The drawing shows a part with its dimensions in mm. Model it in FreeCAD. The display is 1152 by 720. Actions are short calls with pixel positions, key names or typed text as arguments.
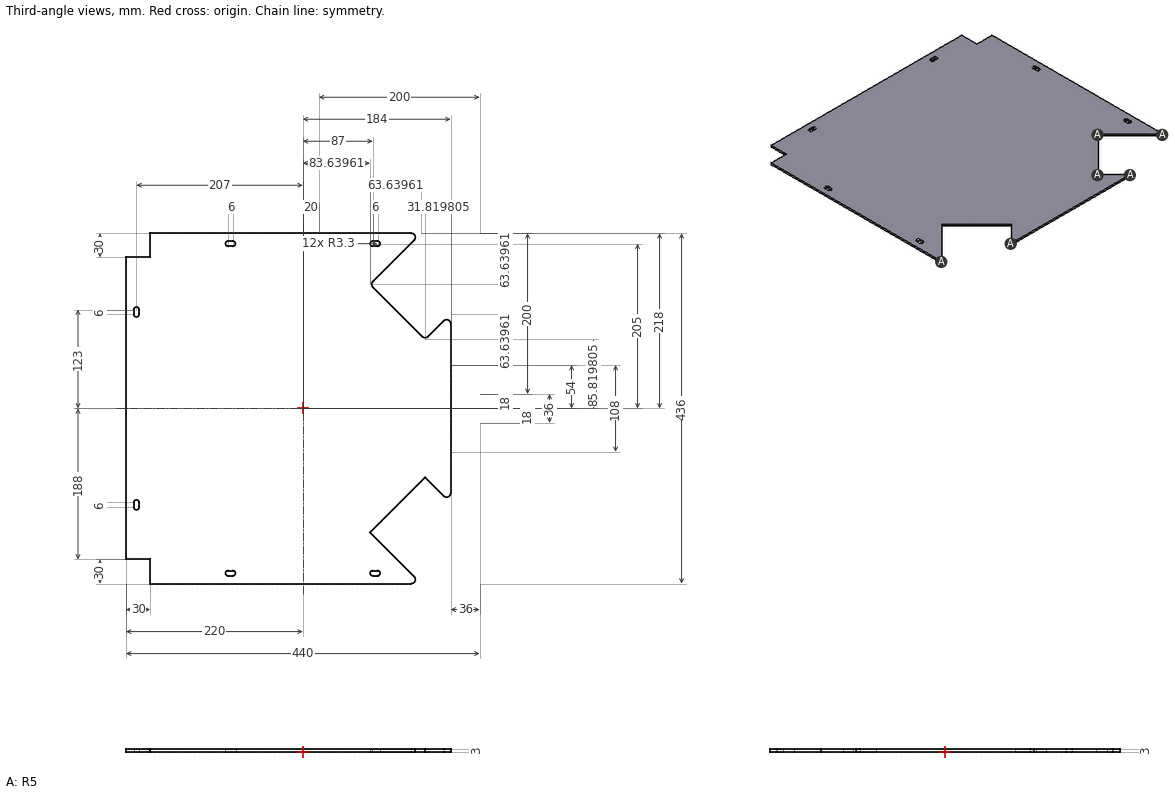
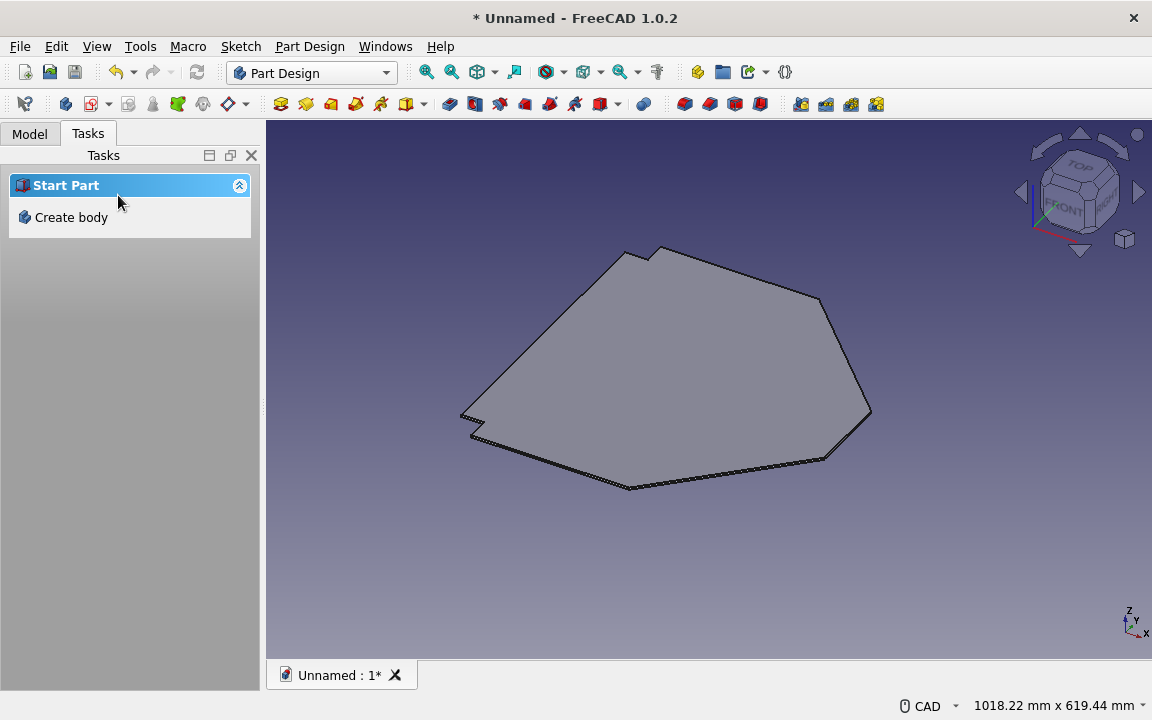
click(695, 383)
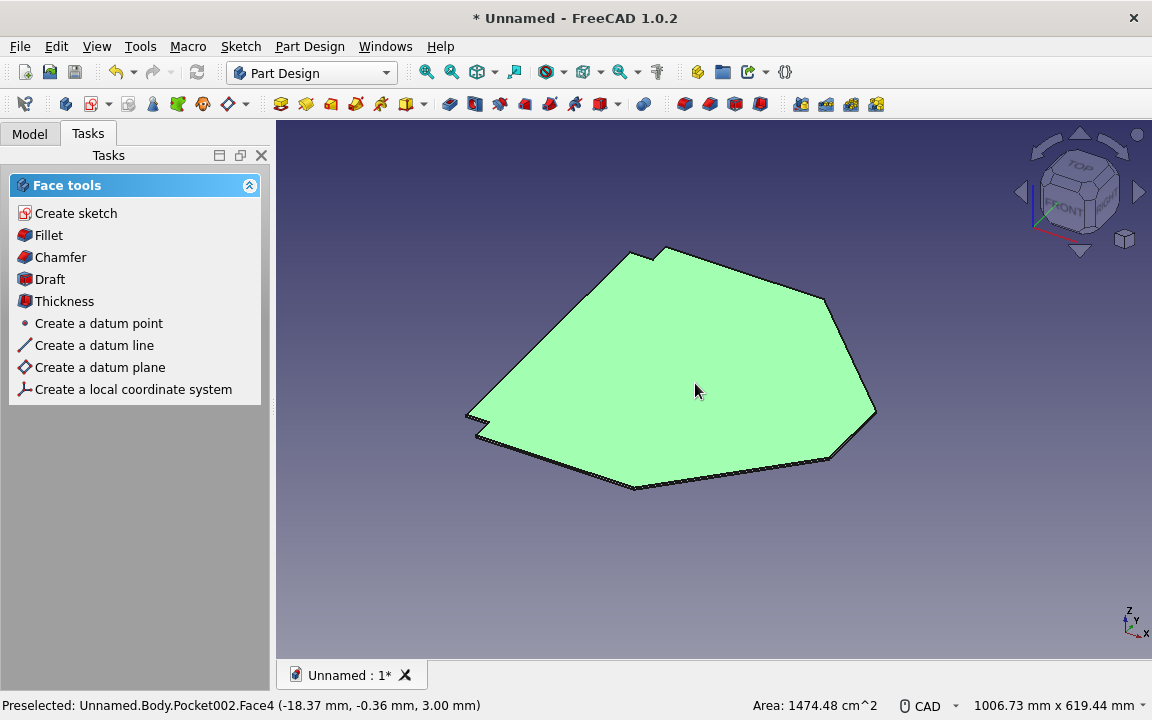
click(90, 104)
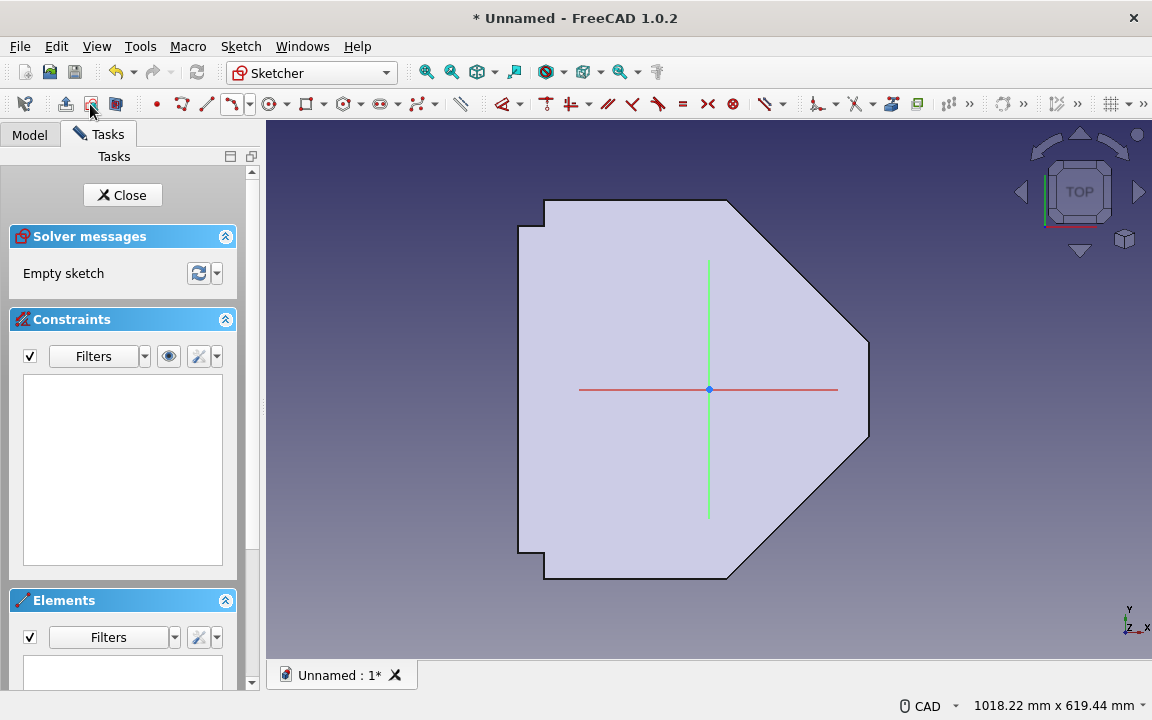
scroll(970, 179, up, 3)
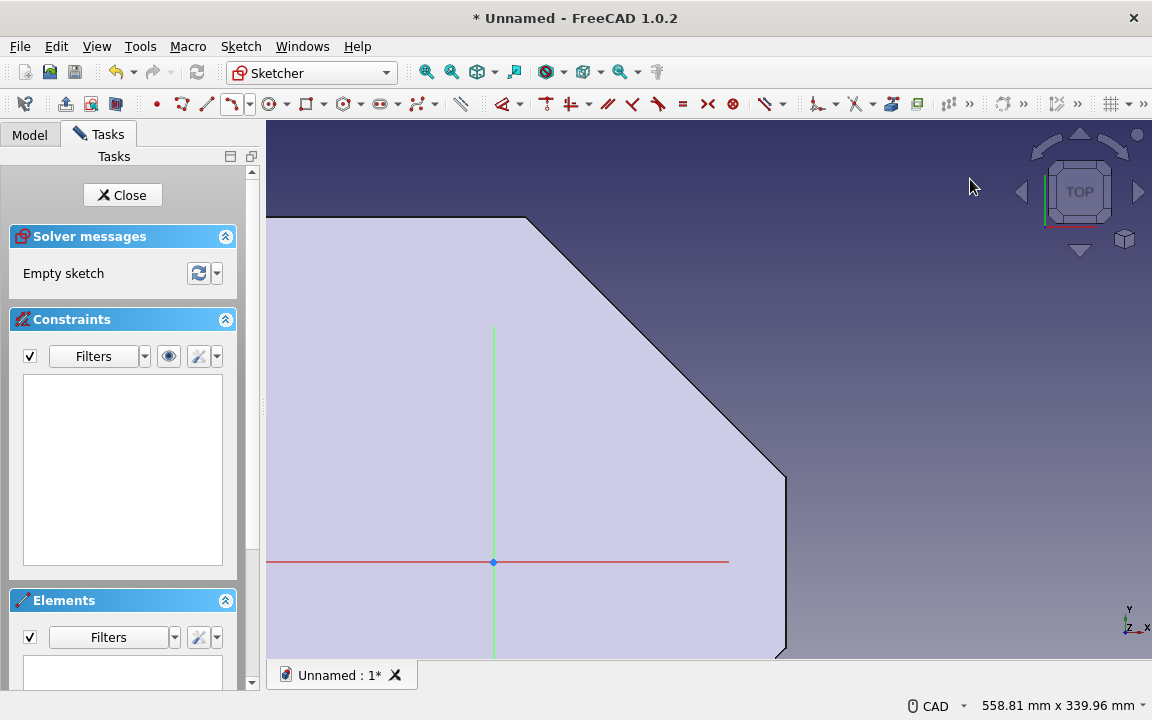
key(g)
key(m)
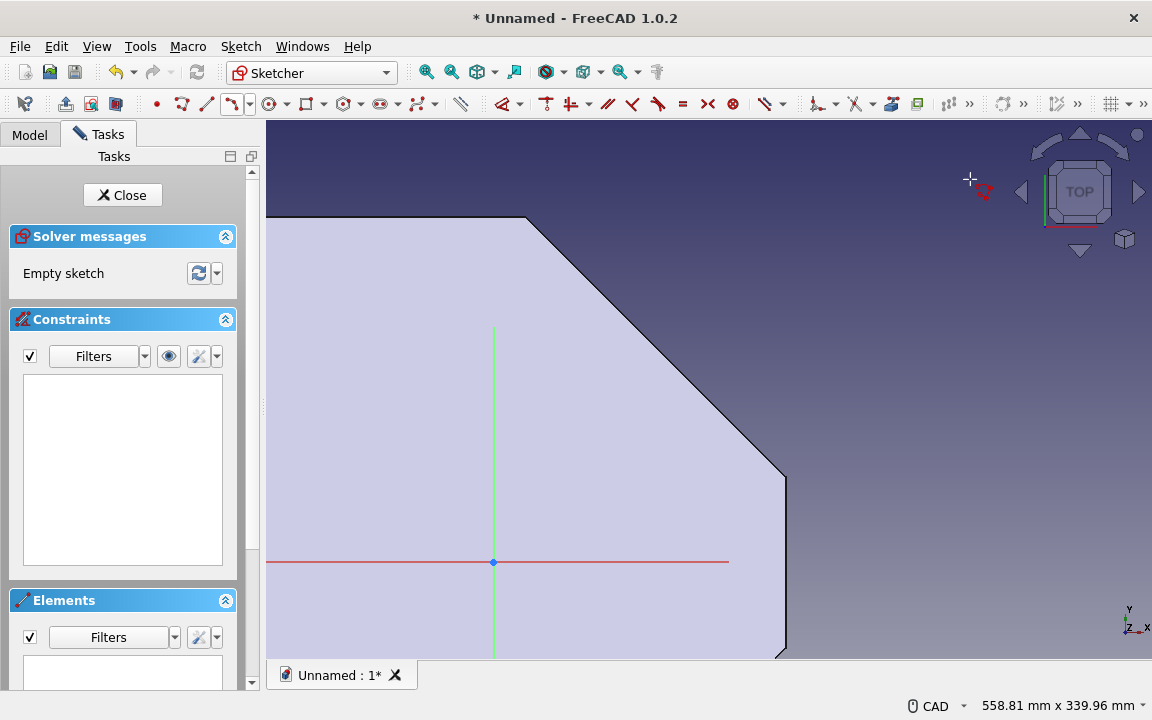
click(626, 318)
click(727, 217)
click(525, 217)
click(626, 319)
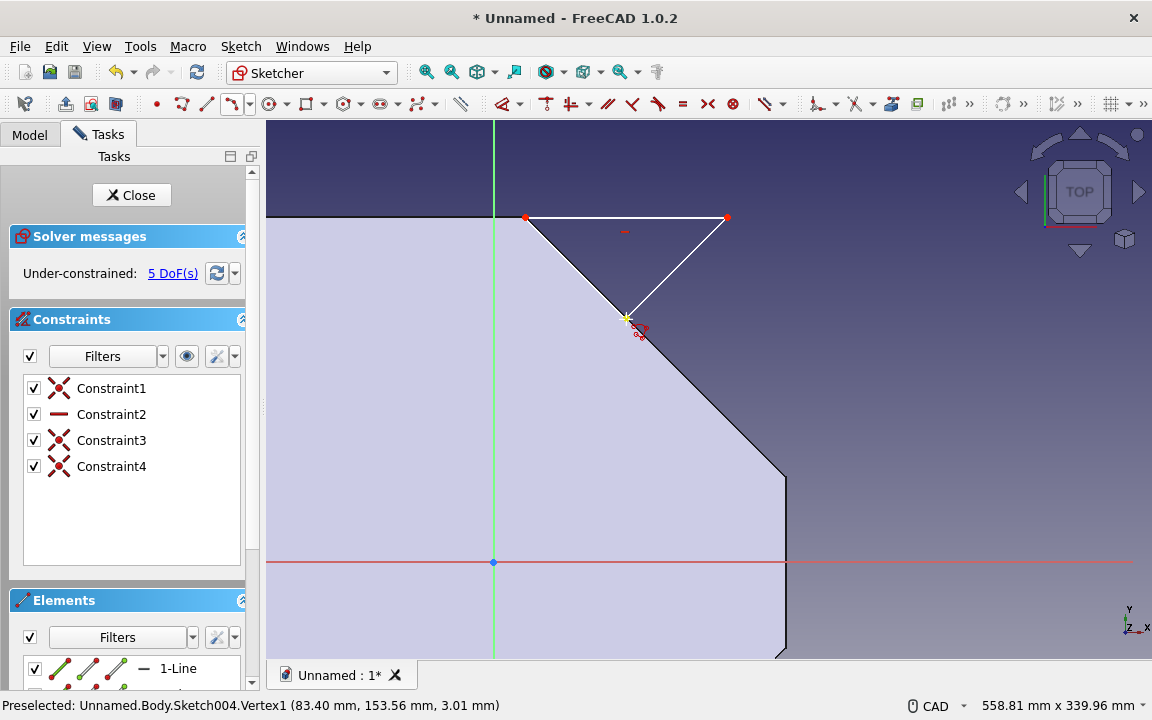
click(735, 426)
click(786, 477)
click(786, 376)
click(735, 427)
key(Escape)
key(Escape)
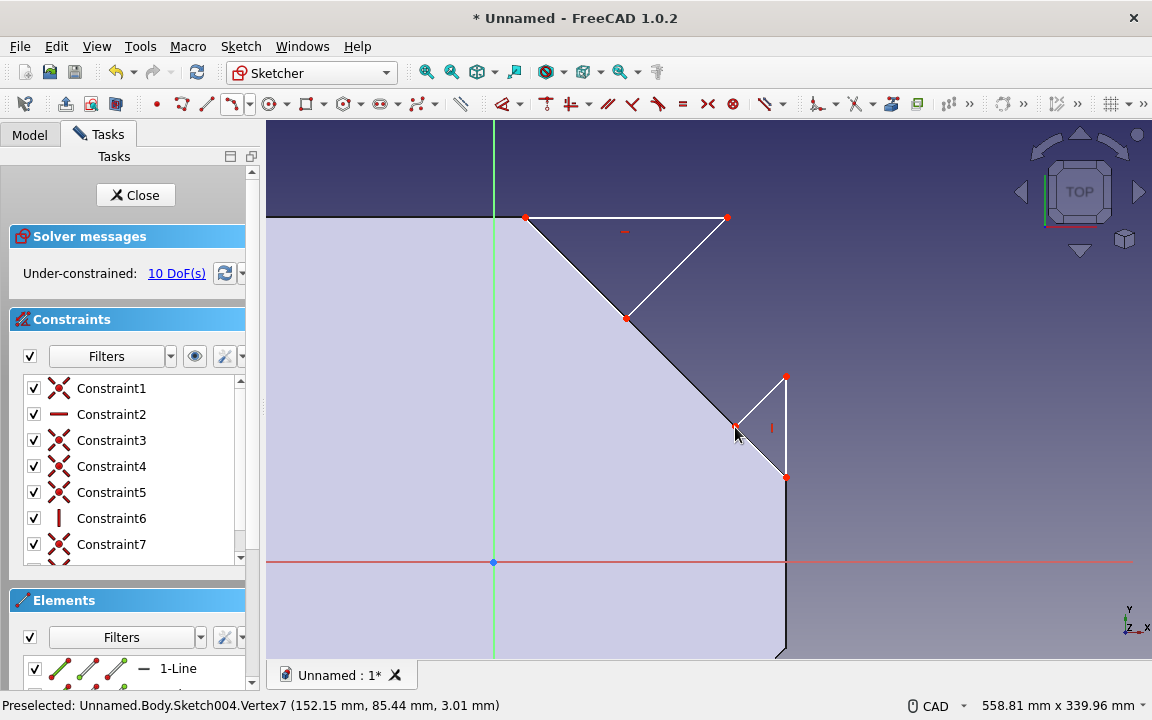
key(d)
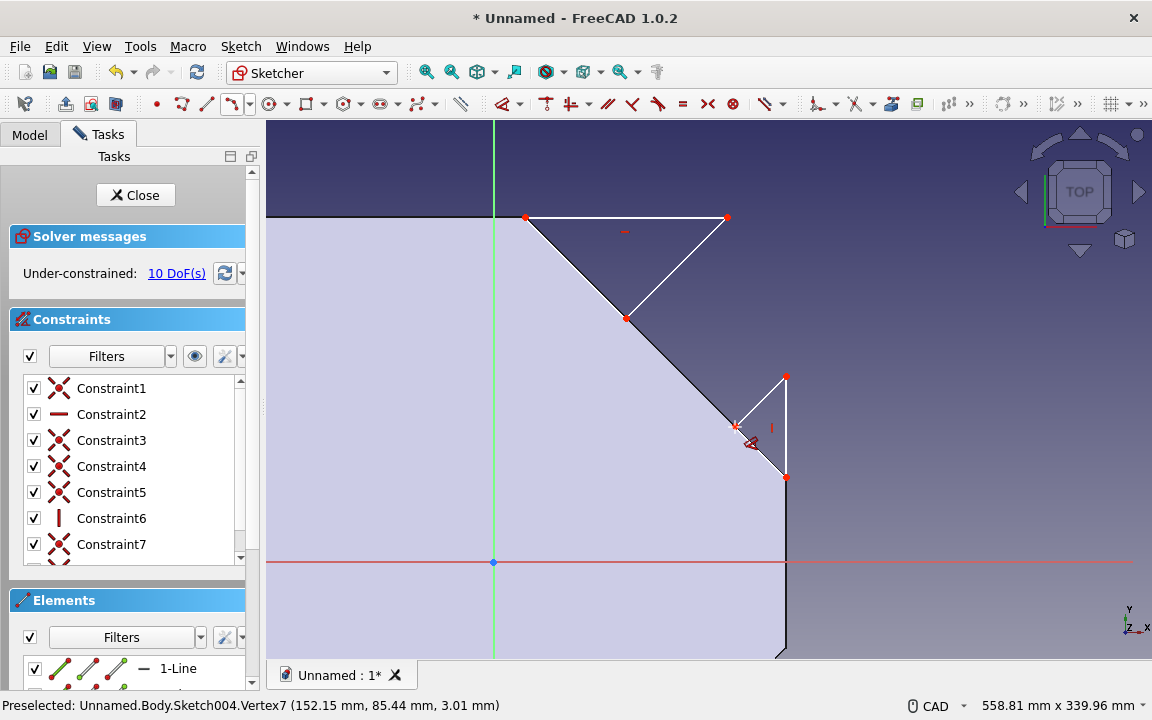
scroll(525, 218, up, 2)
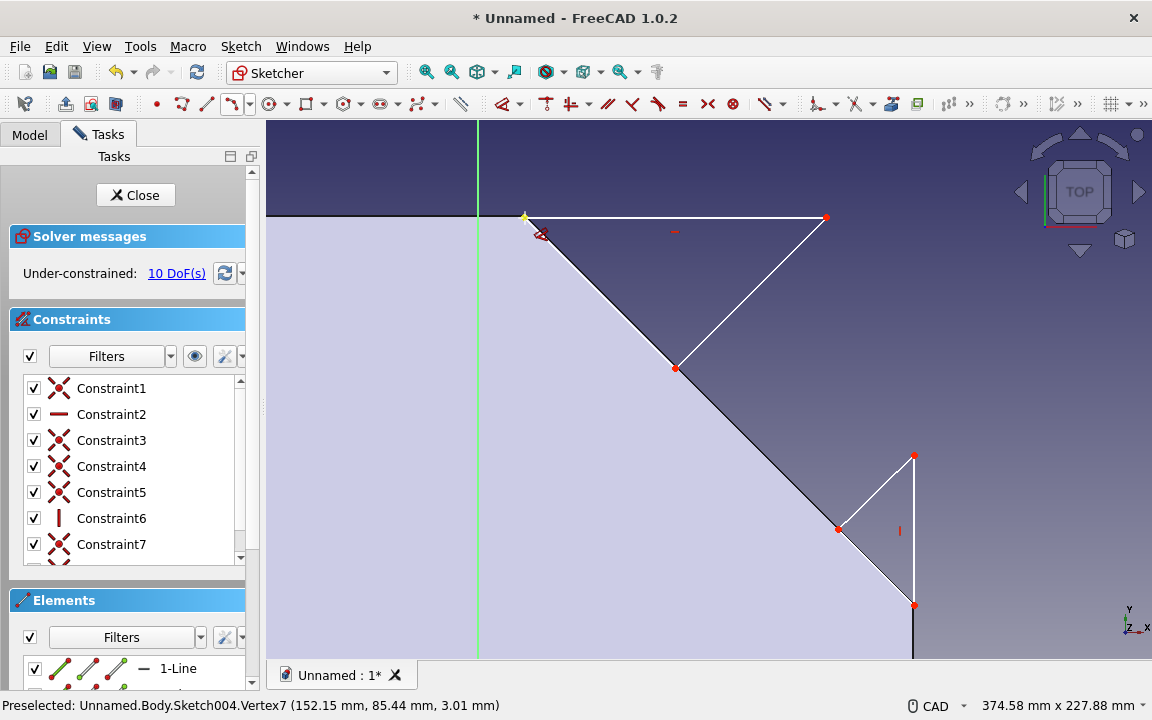
click(525, 218)
click(502, 184)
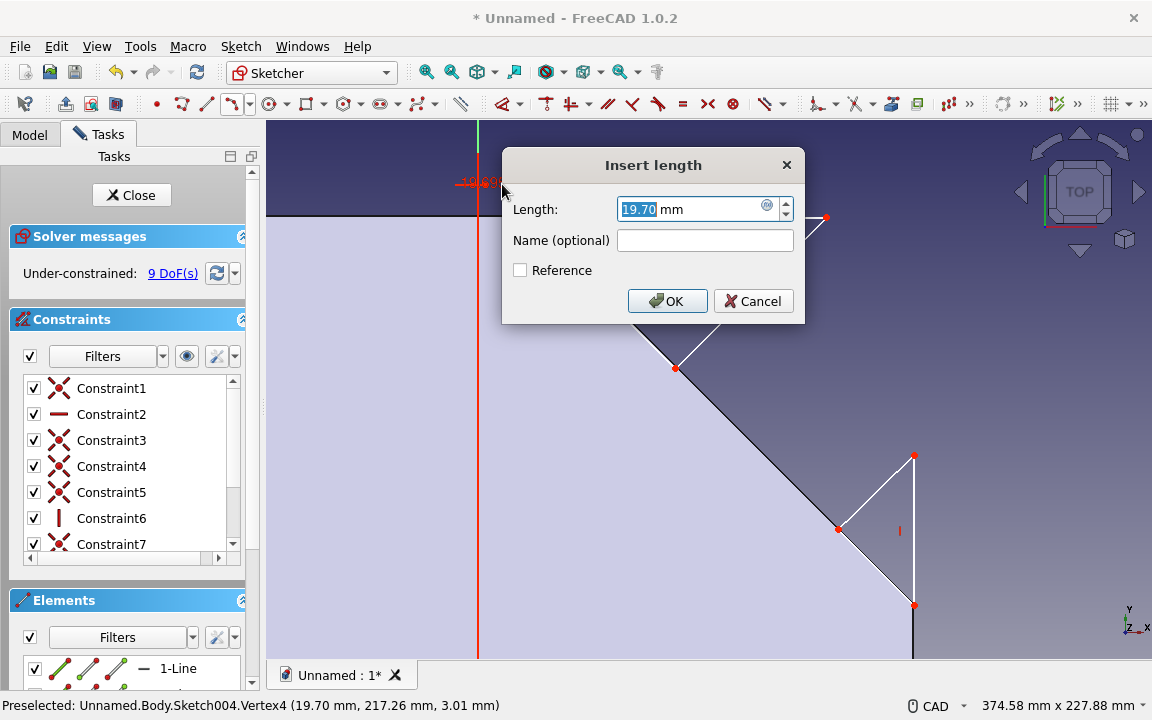
text(20)
key(Return)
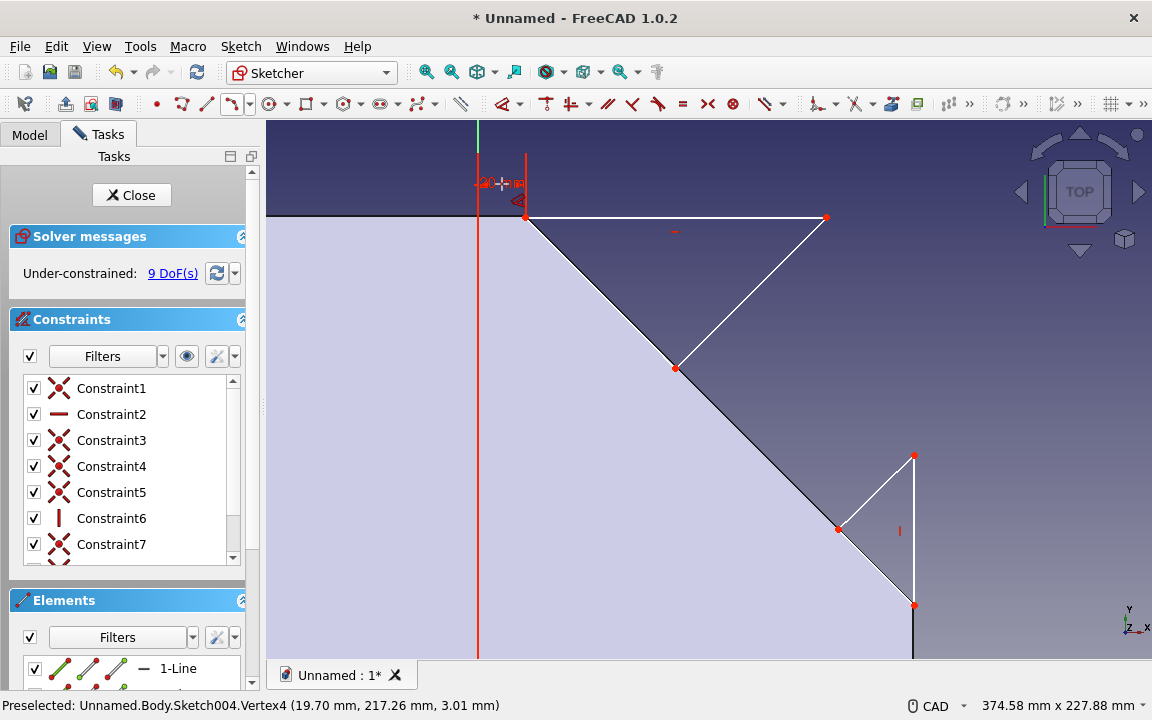
click(914, 606)
click(948, 618)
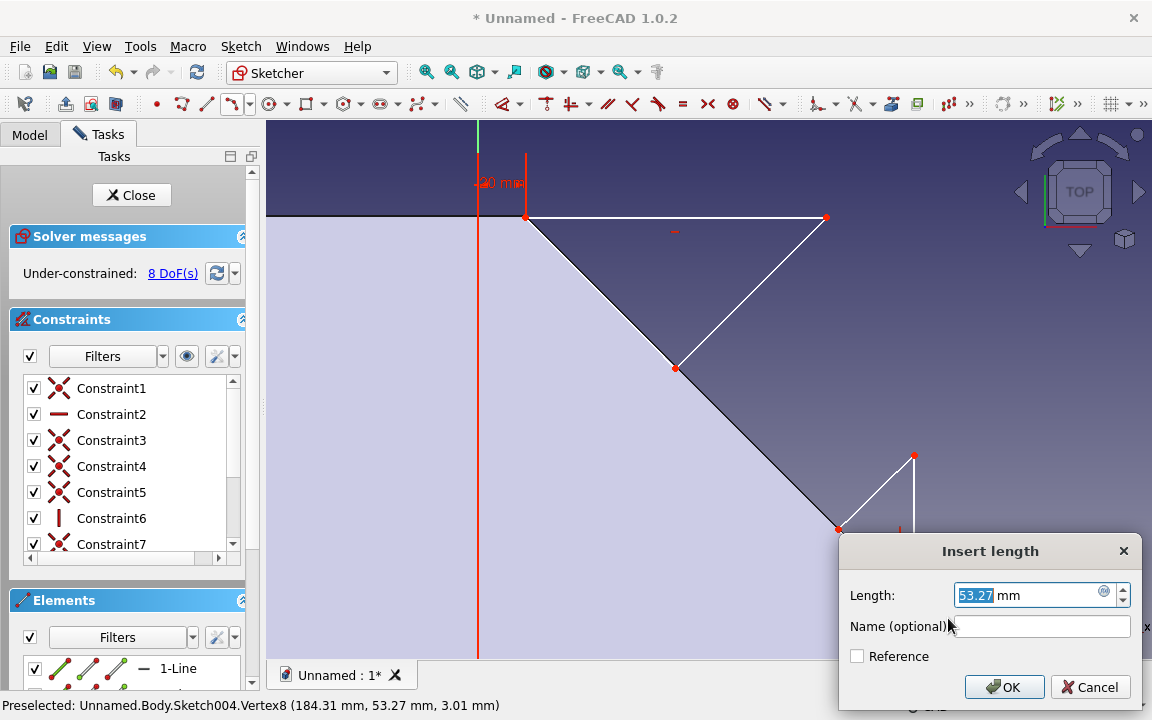
text(54)
key(Return)